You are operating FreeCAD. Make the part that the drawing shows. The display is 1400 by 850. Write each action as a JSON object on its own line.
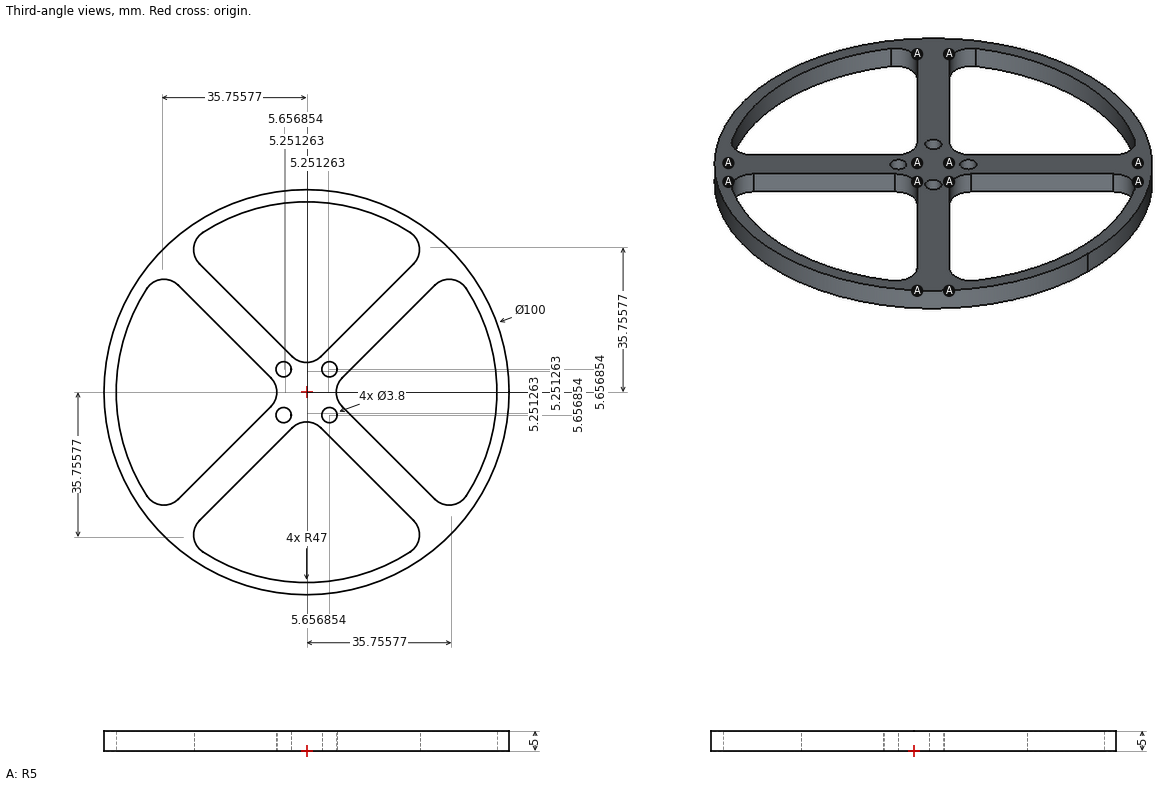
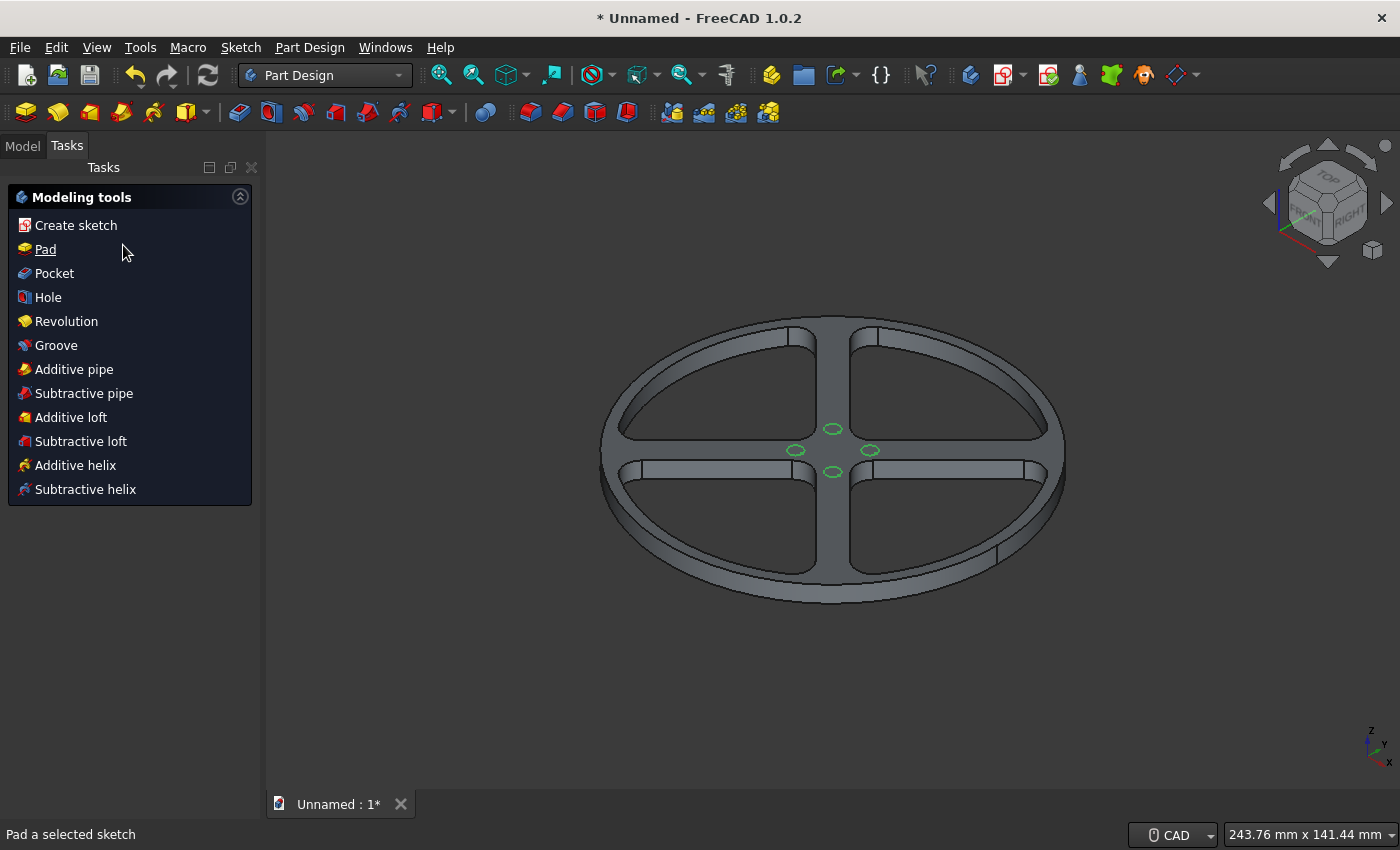
{"action": "left_click", "coordinate": [240, 112]}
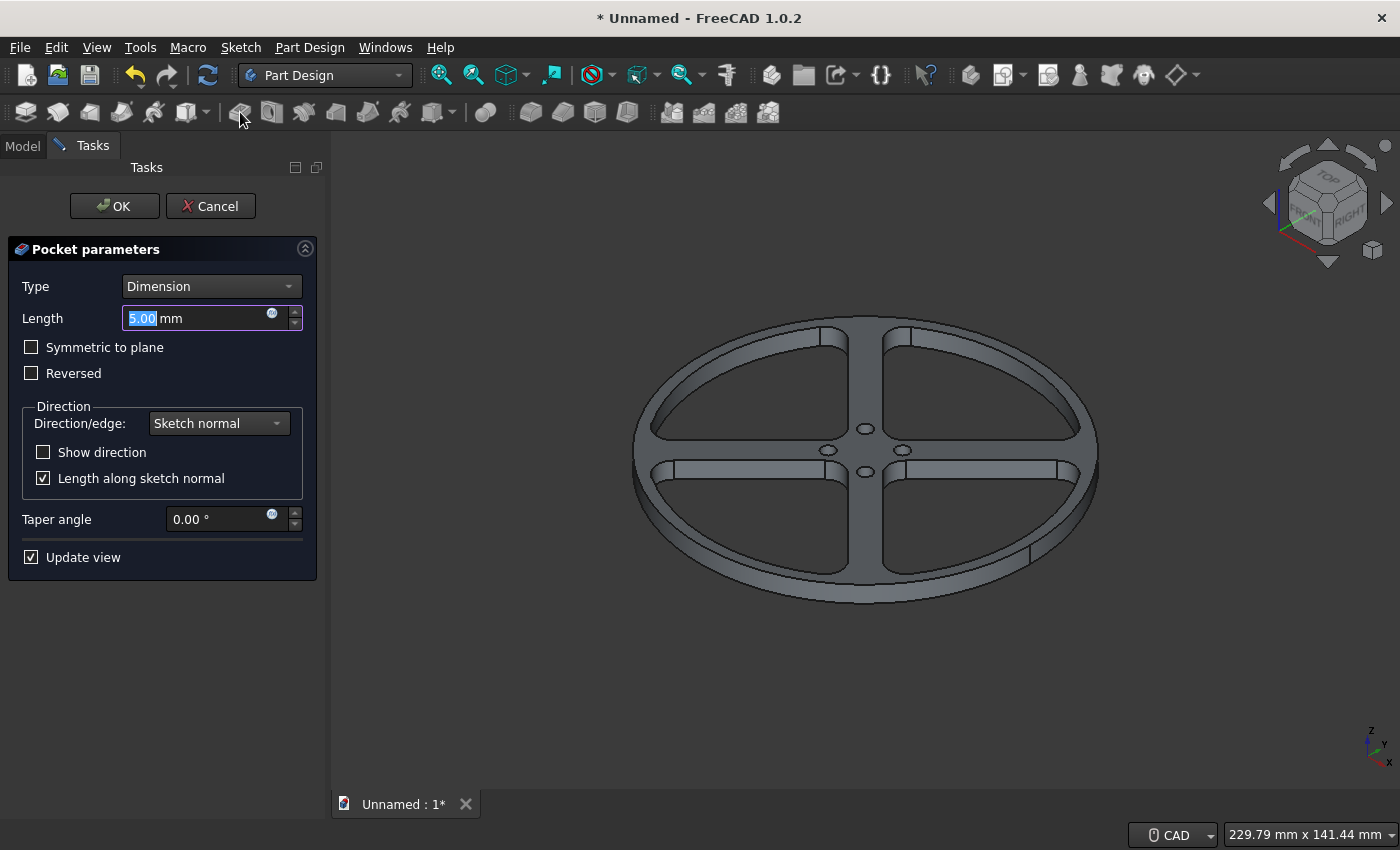
{"action": "type", "text": "5"}
{"action": "key", "text": "Tab"}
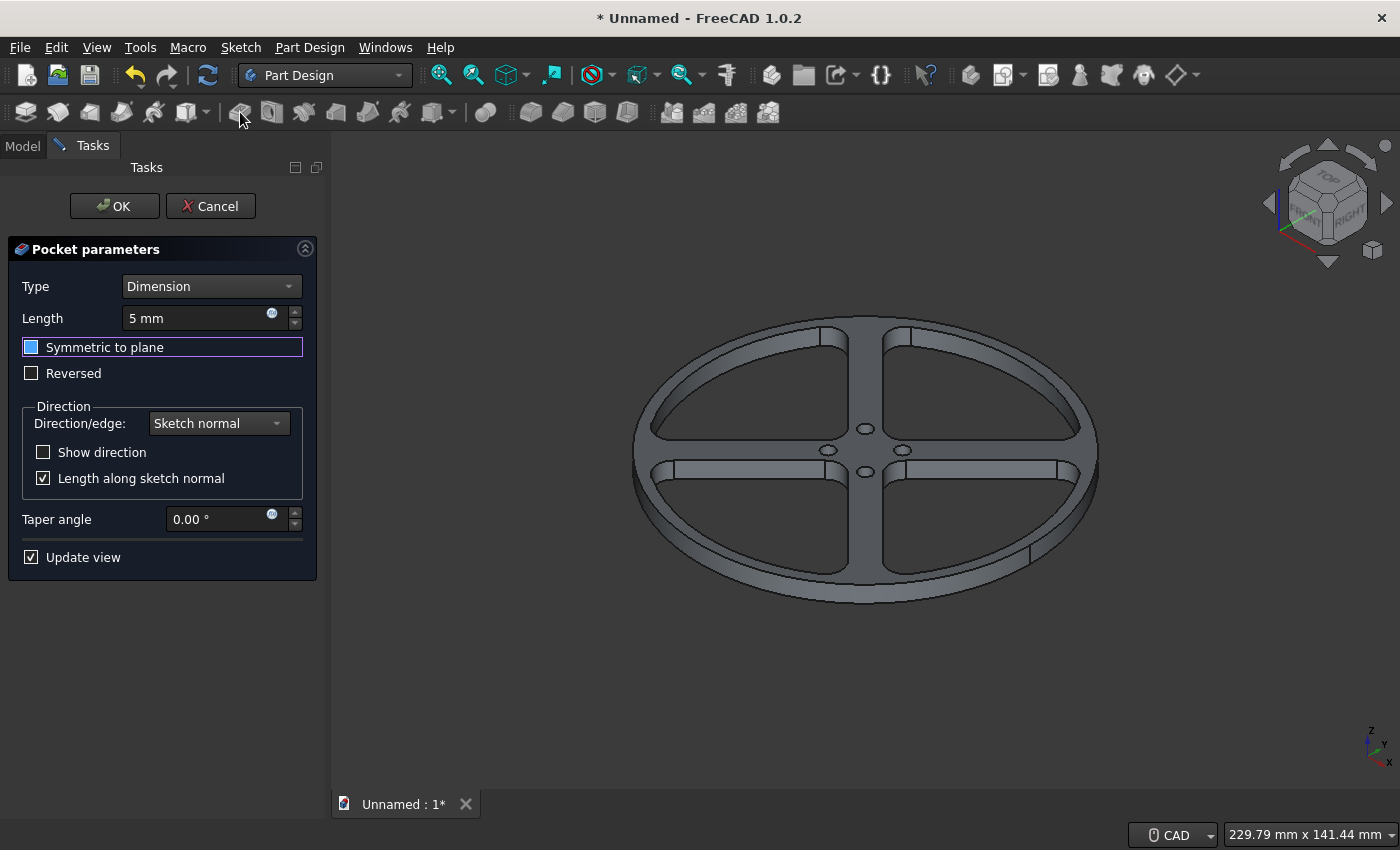
{"action": "left_click", "coordinate": [115, 206]}